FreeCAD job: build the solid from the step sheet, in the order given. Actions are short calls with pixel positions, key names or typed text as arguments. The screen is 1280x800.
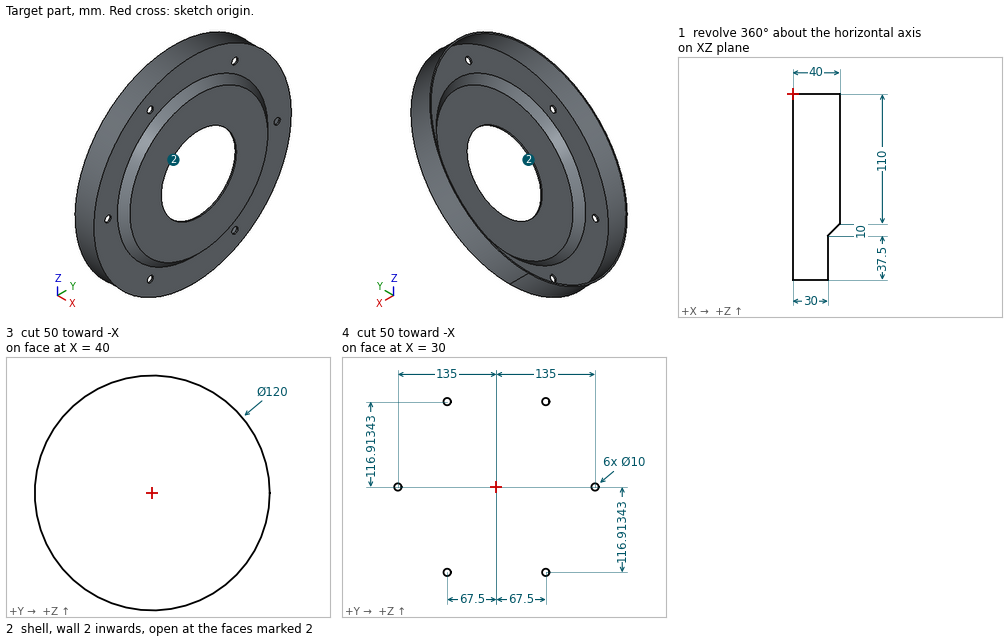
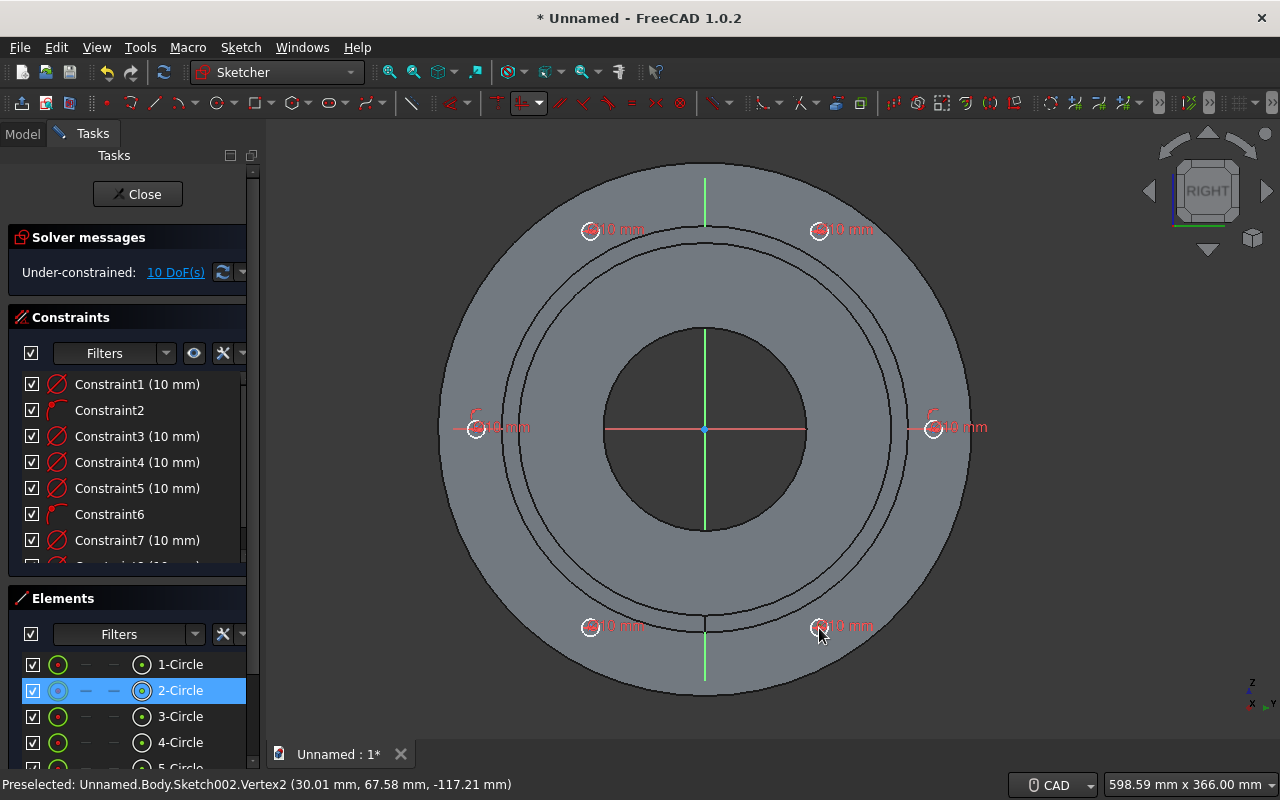
click(590, 628)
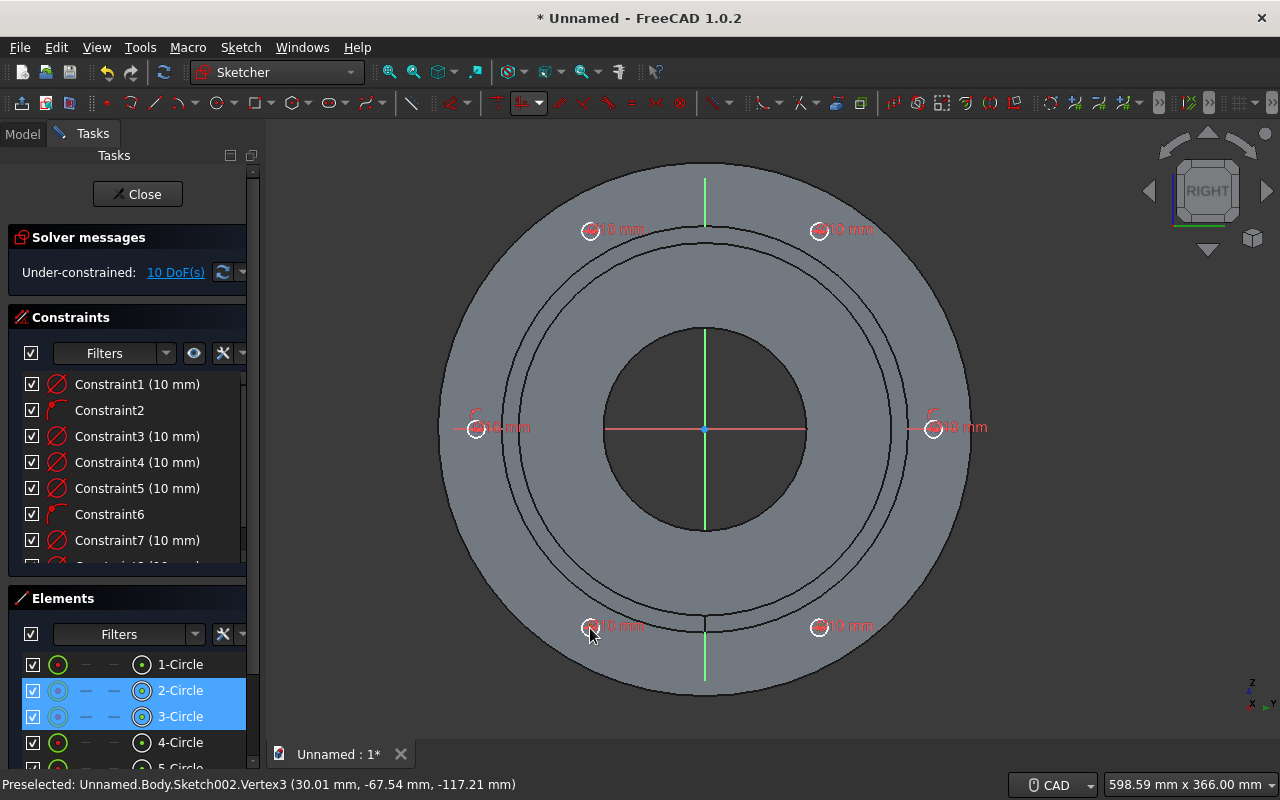
click(542, 104)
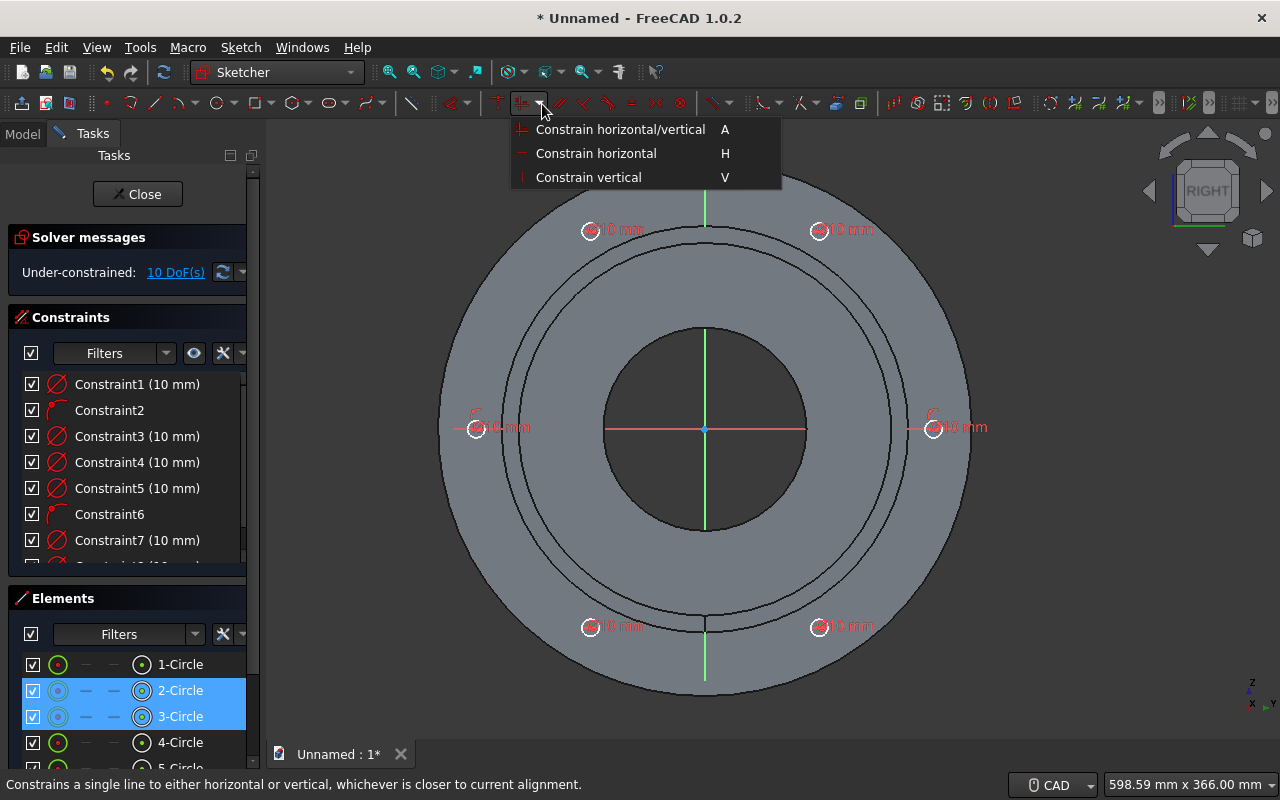
click(646, 153)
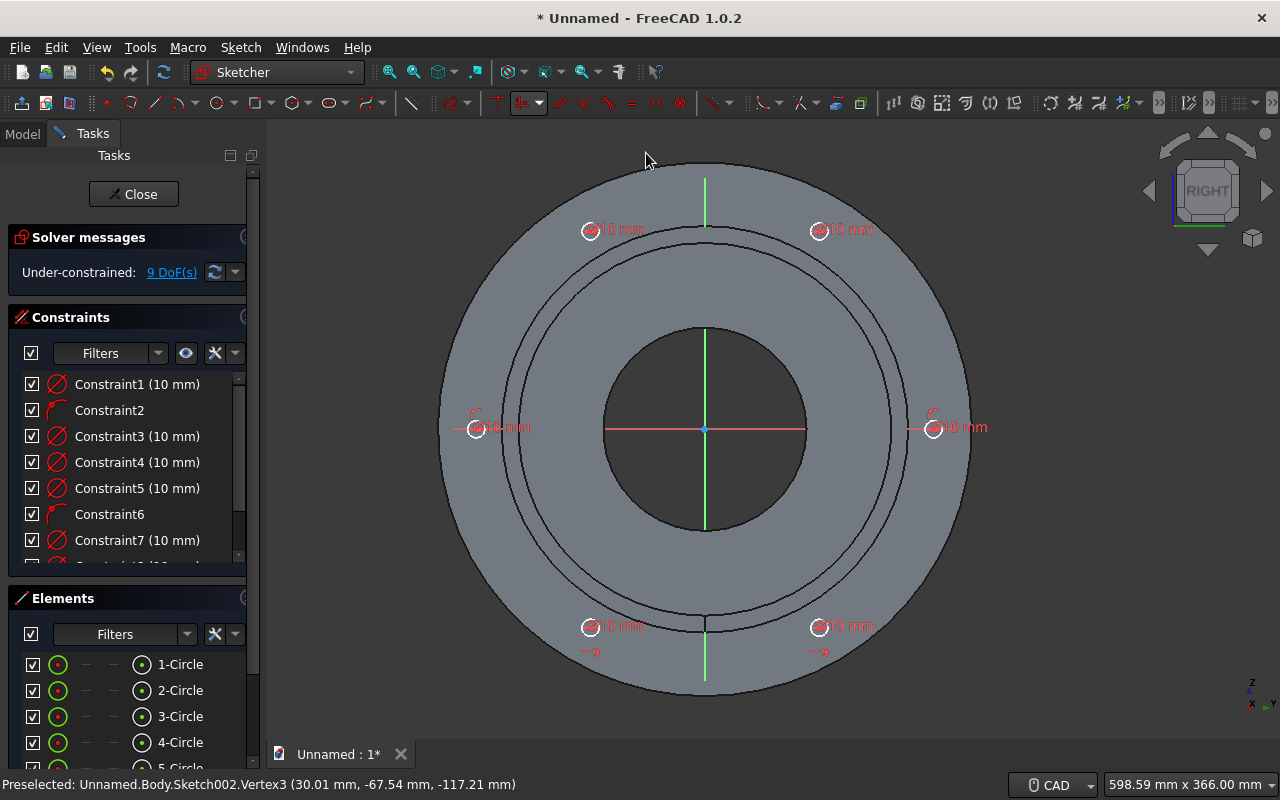
click(590, 628)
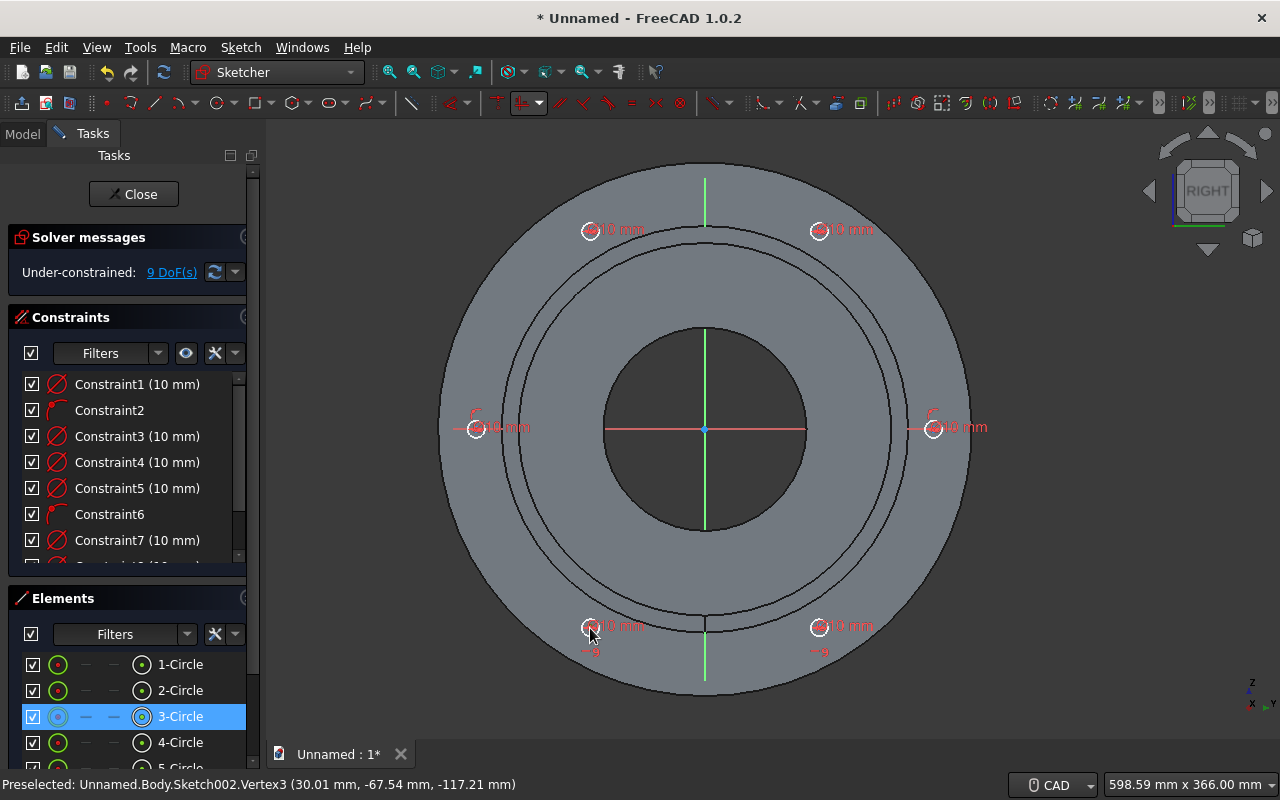
click(590, 231)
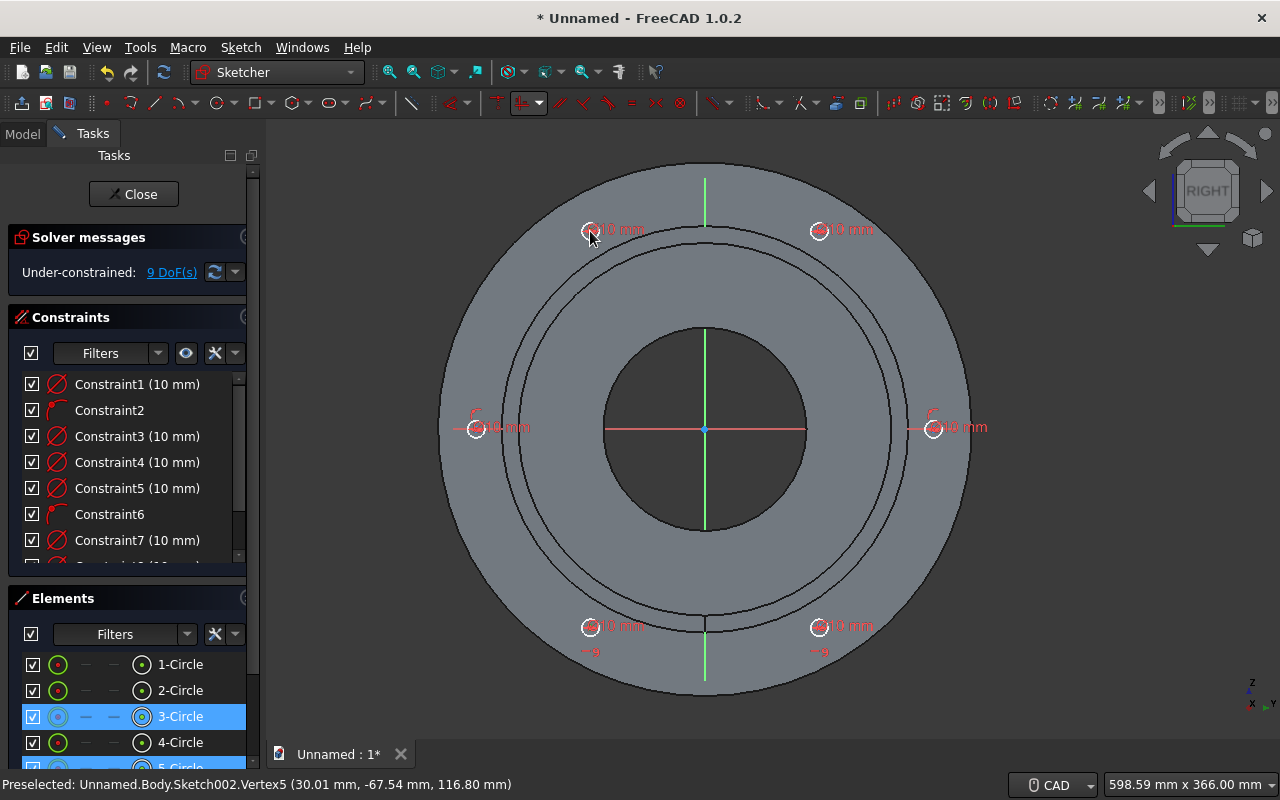
key(v)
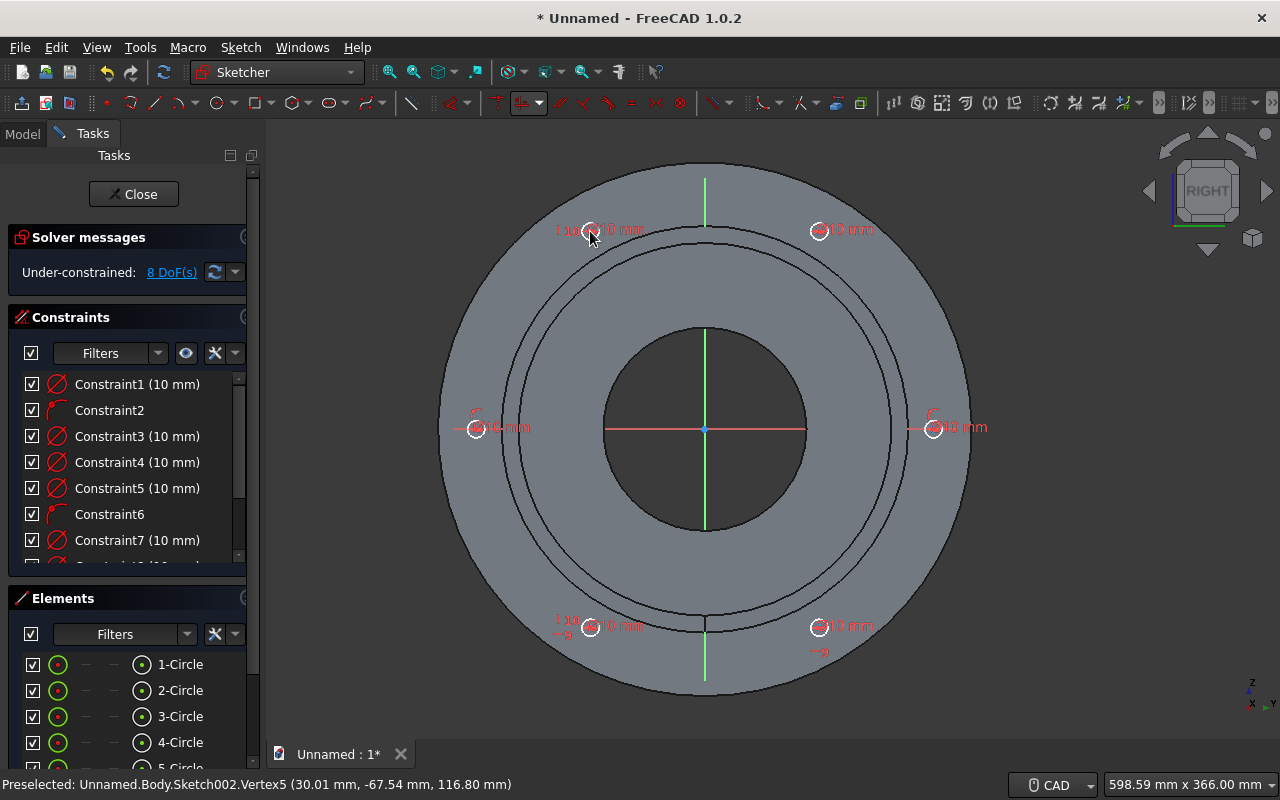
click(819, 628)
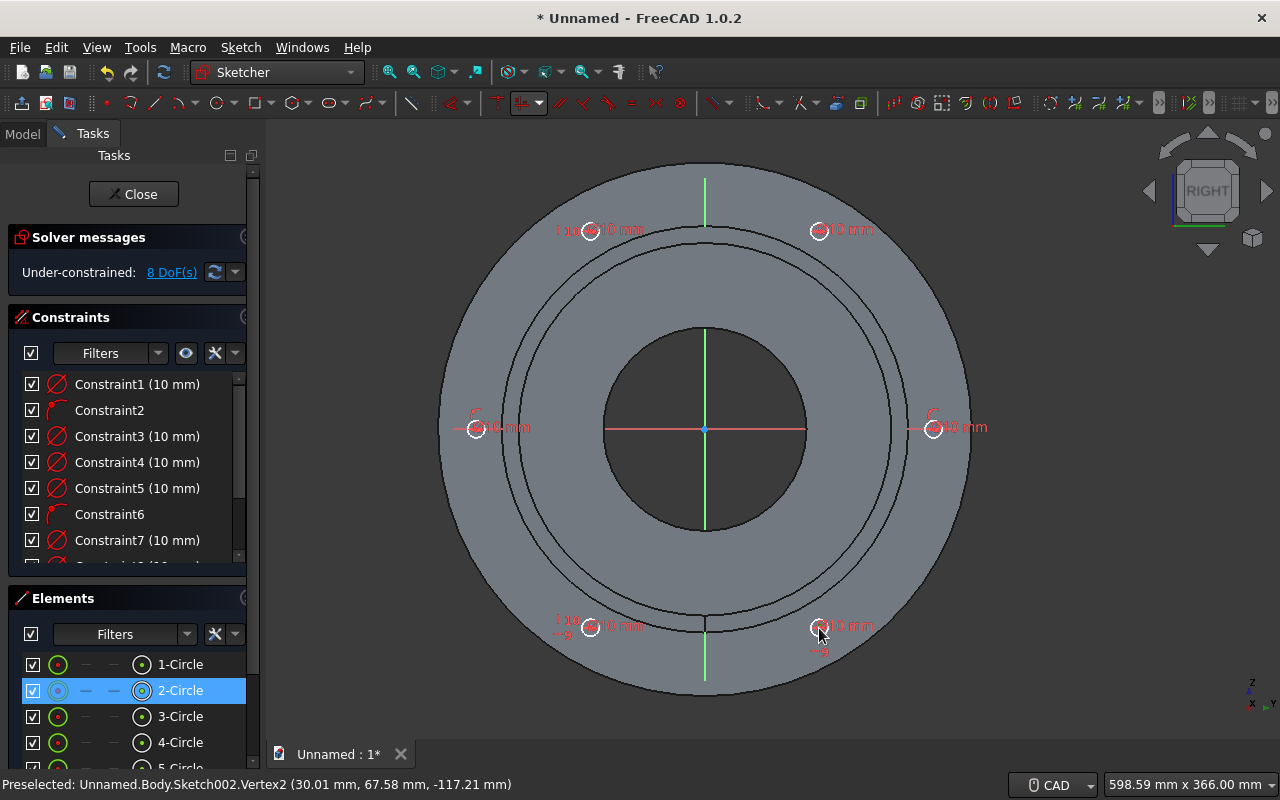
click(819, 231)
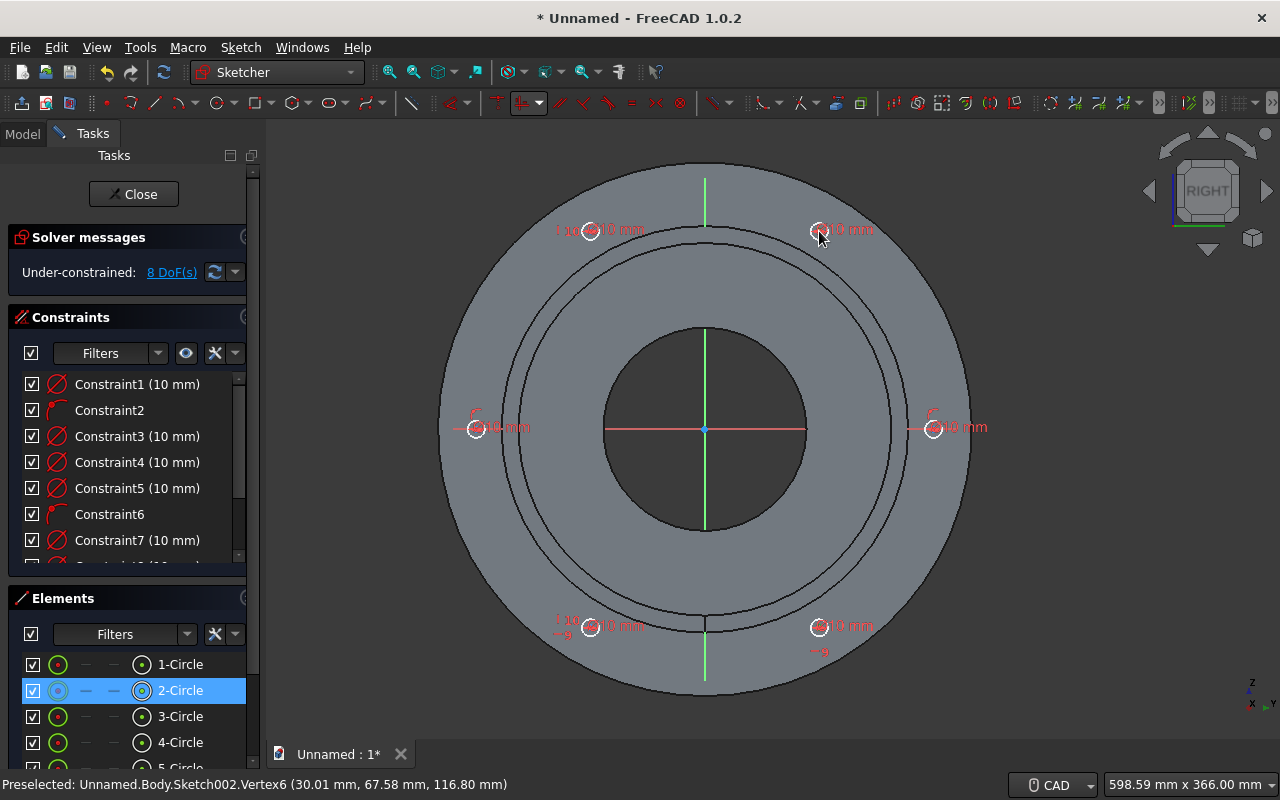
key(v)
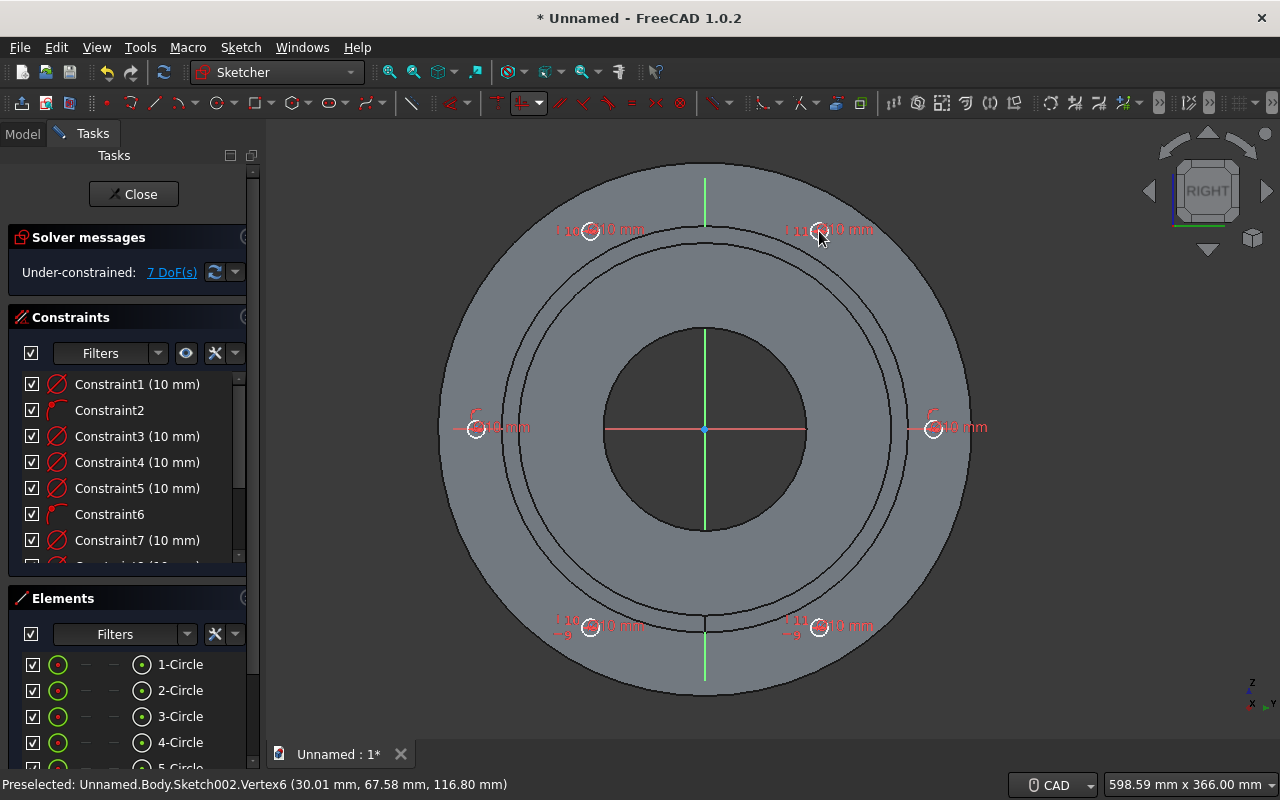
click(590, 231)